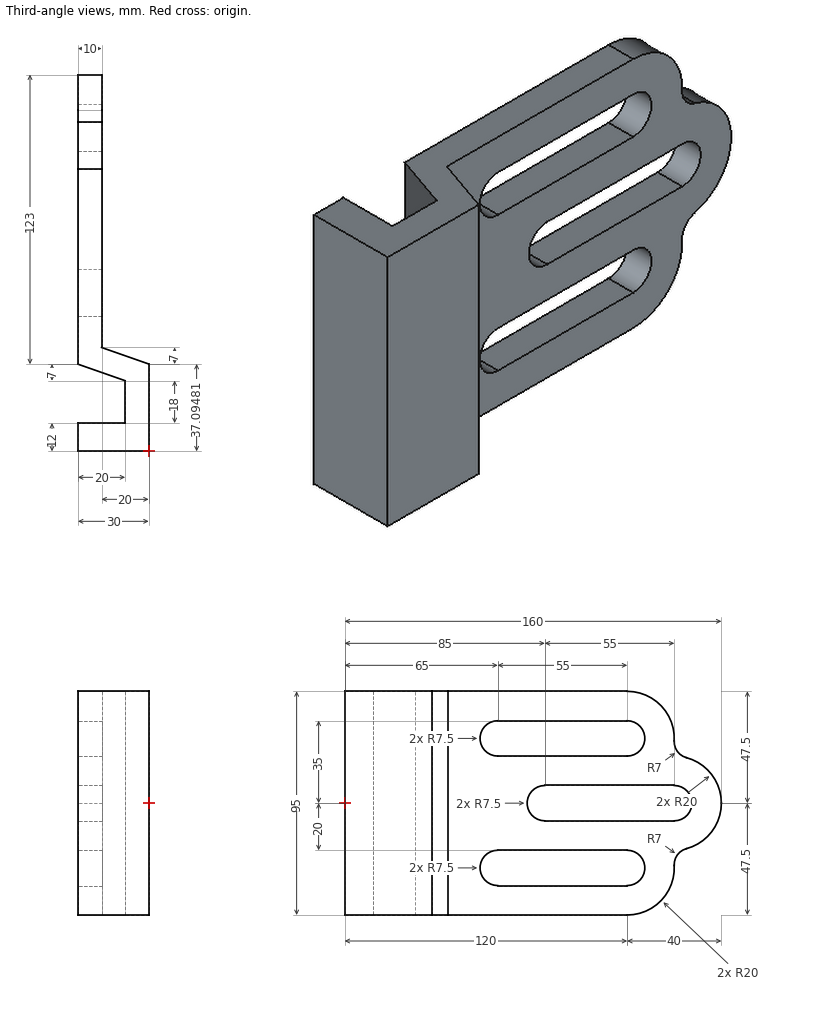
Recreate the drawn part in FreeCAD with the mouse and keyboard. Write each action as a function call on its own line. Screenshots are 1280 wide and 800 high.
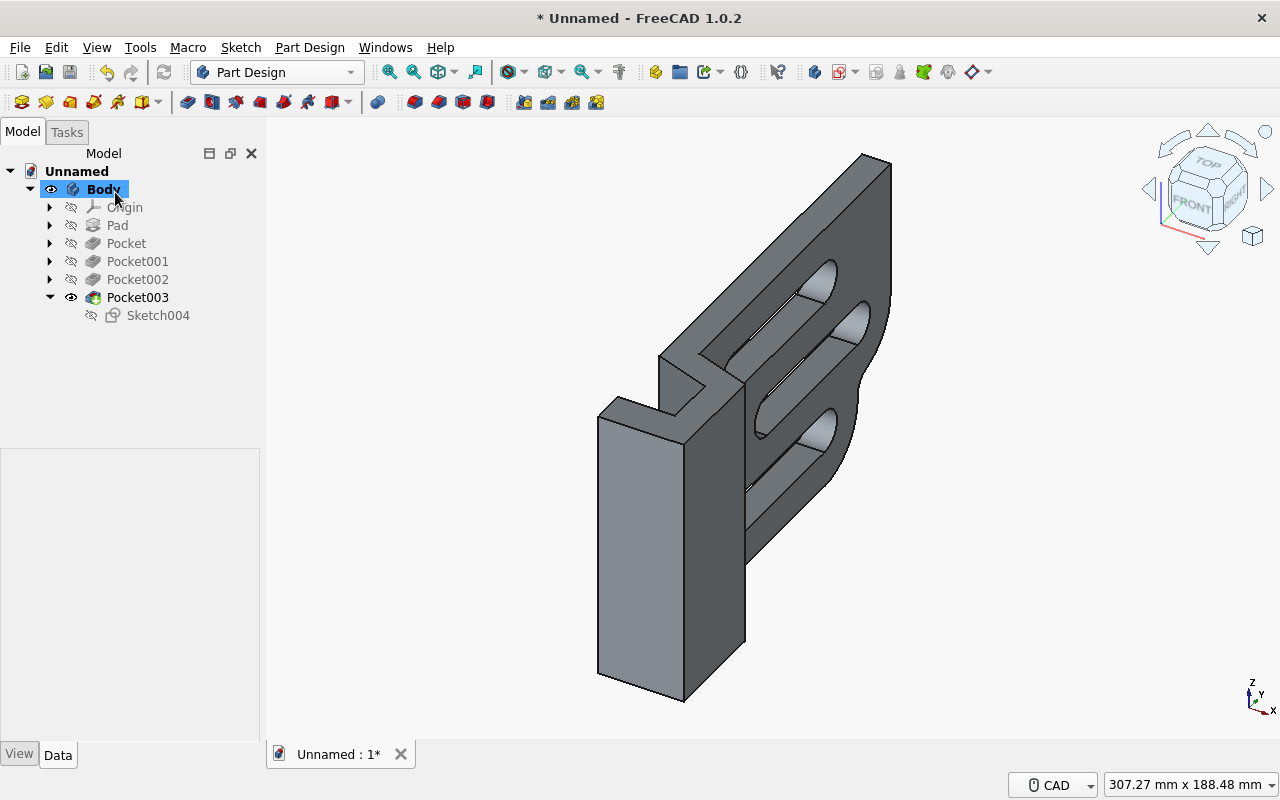
click(877, 231)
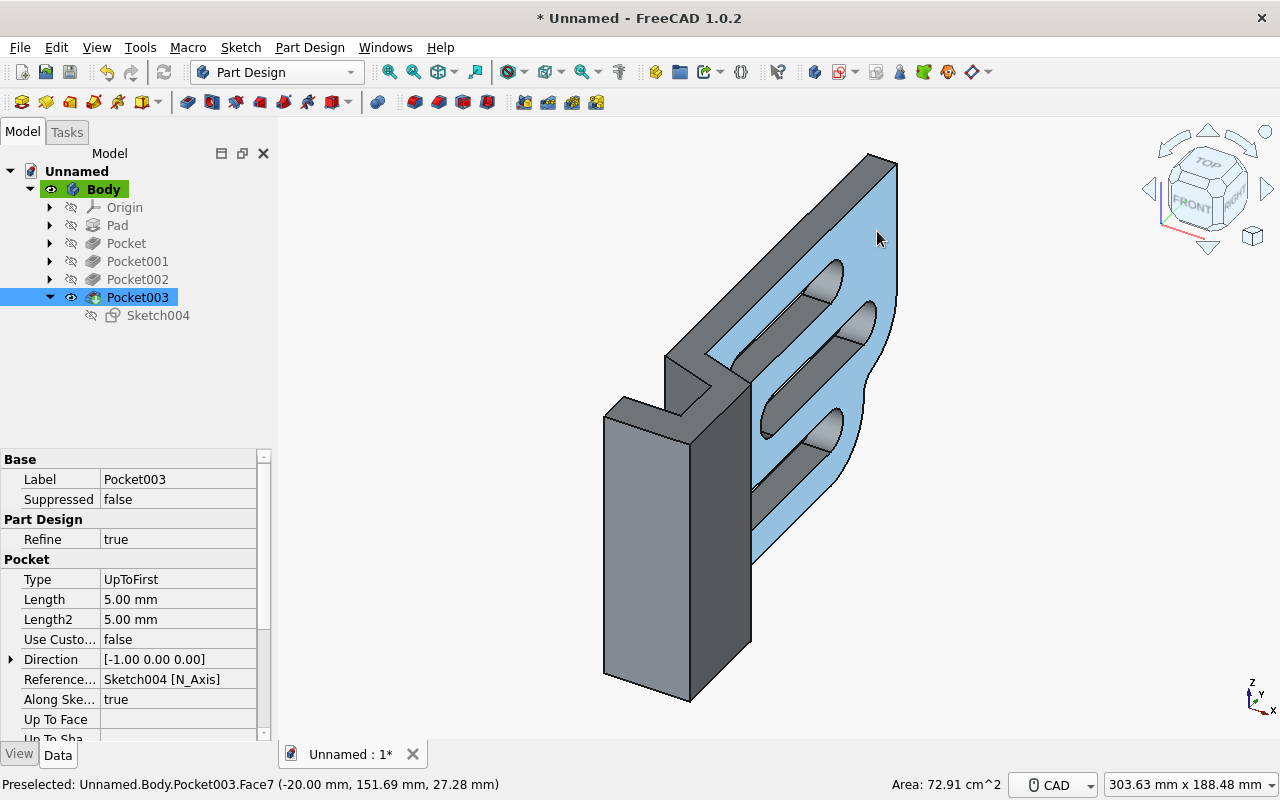
click(840, 72)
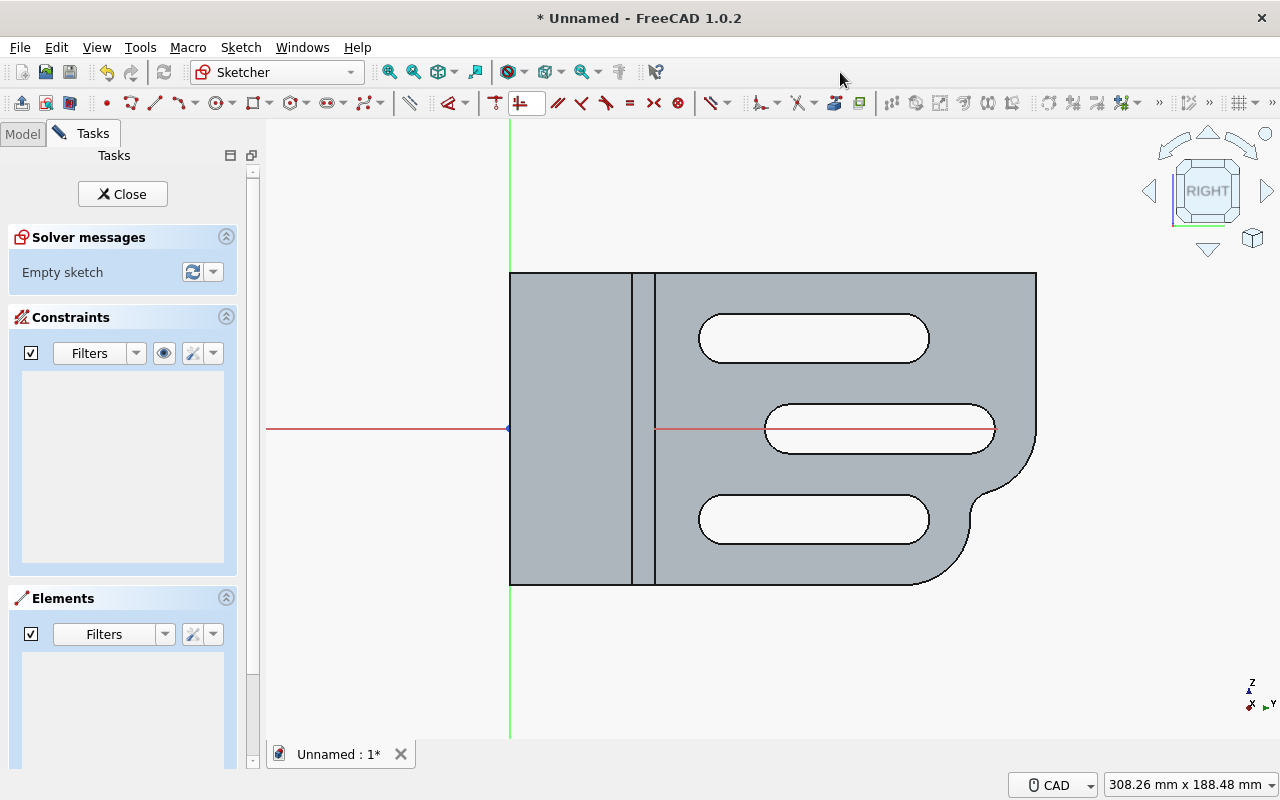
click(70, 104)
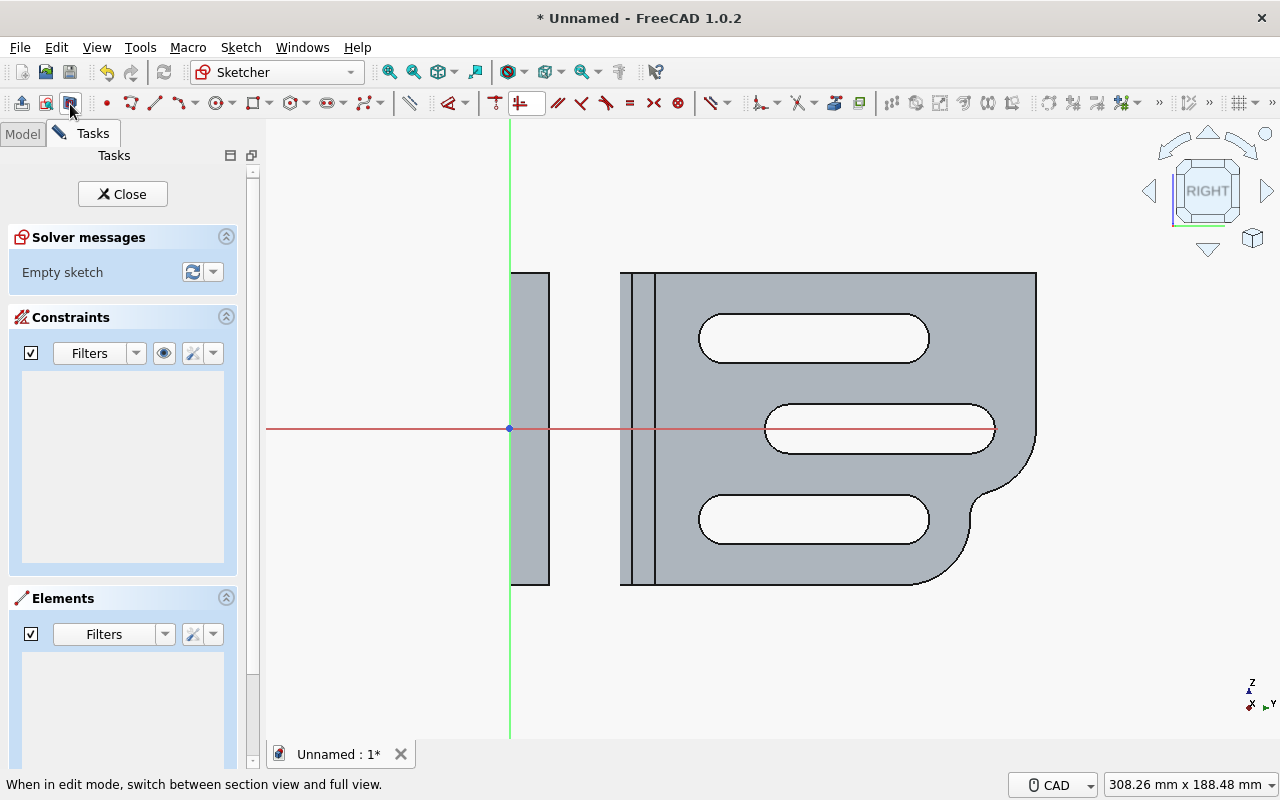
scroll(1115, 305, up, 5)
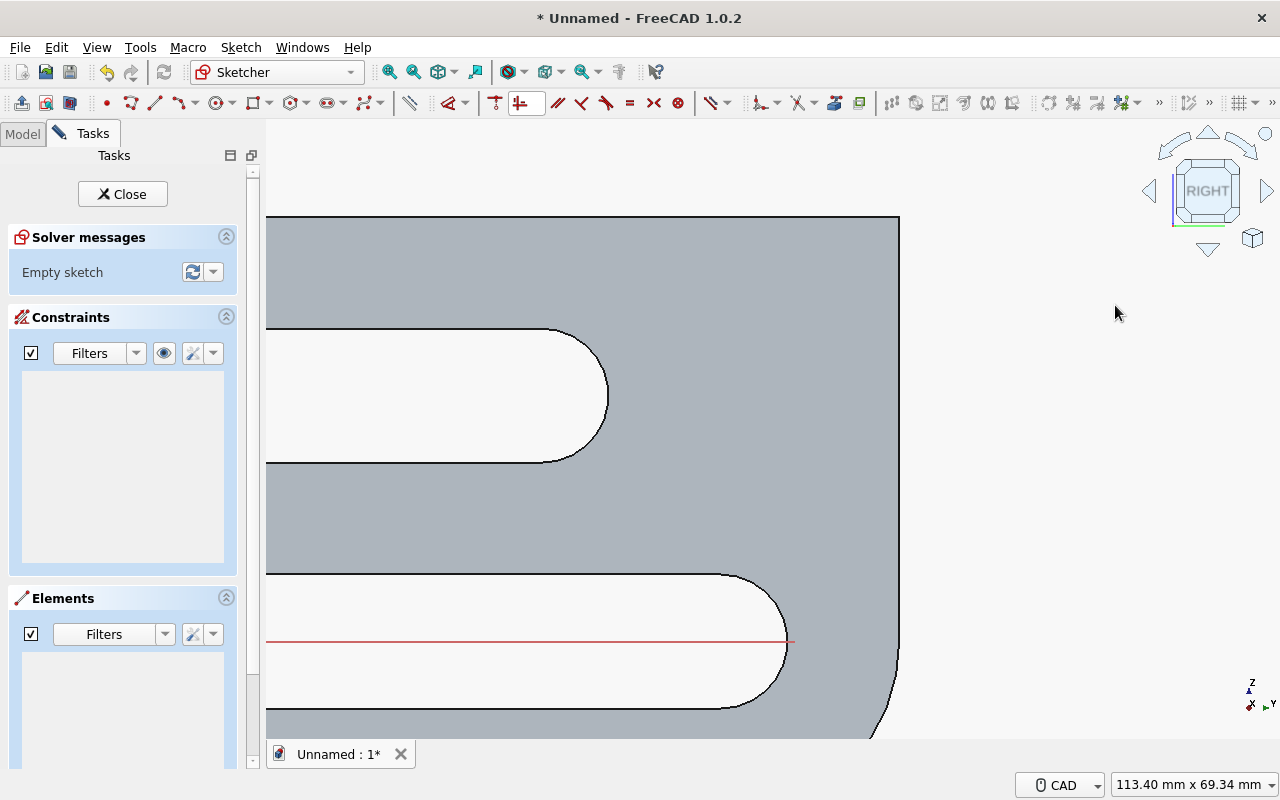
click(132, 104)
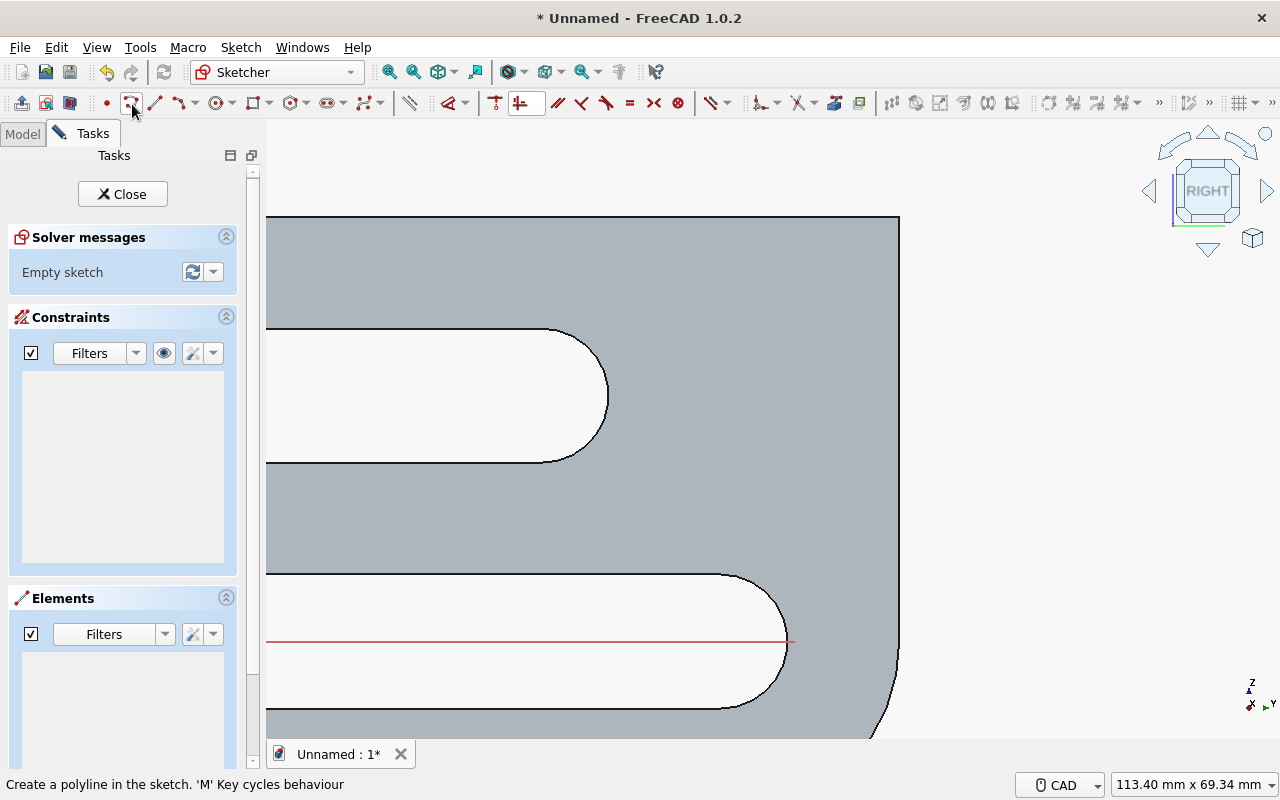
click(899, 642)
click(899, 217)
click(542, 217)
right_click(542, 217)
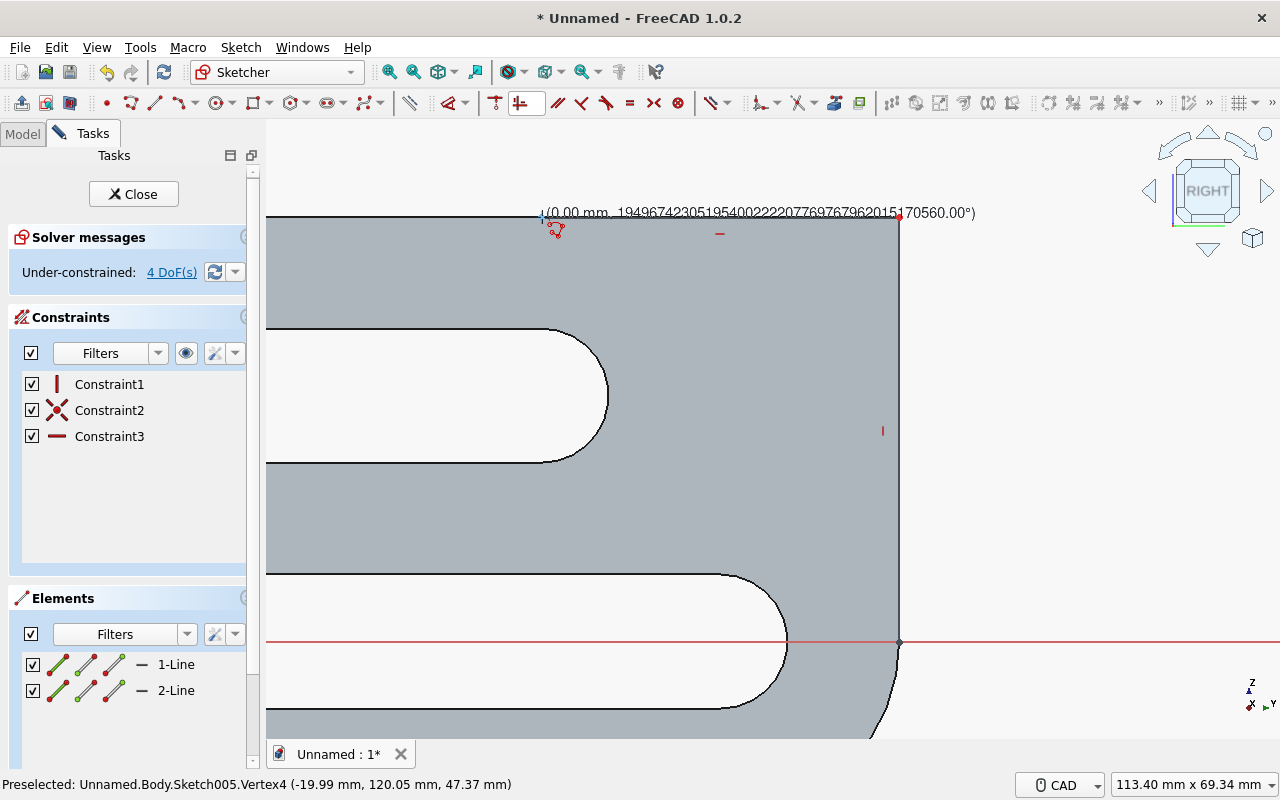
click(180, 104)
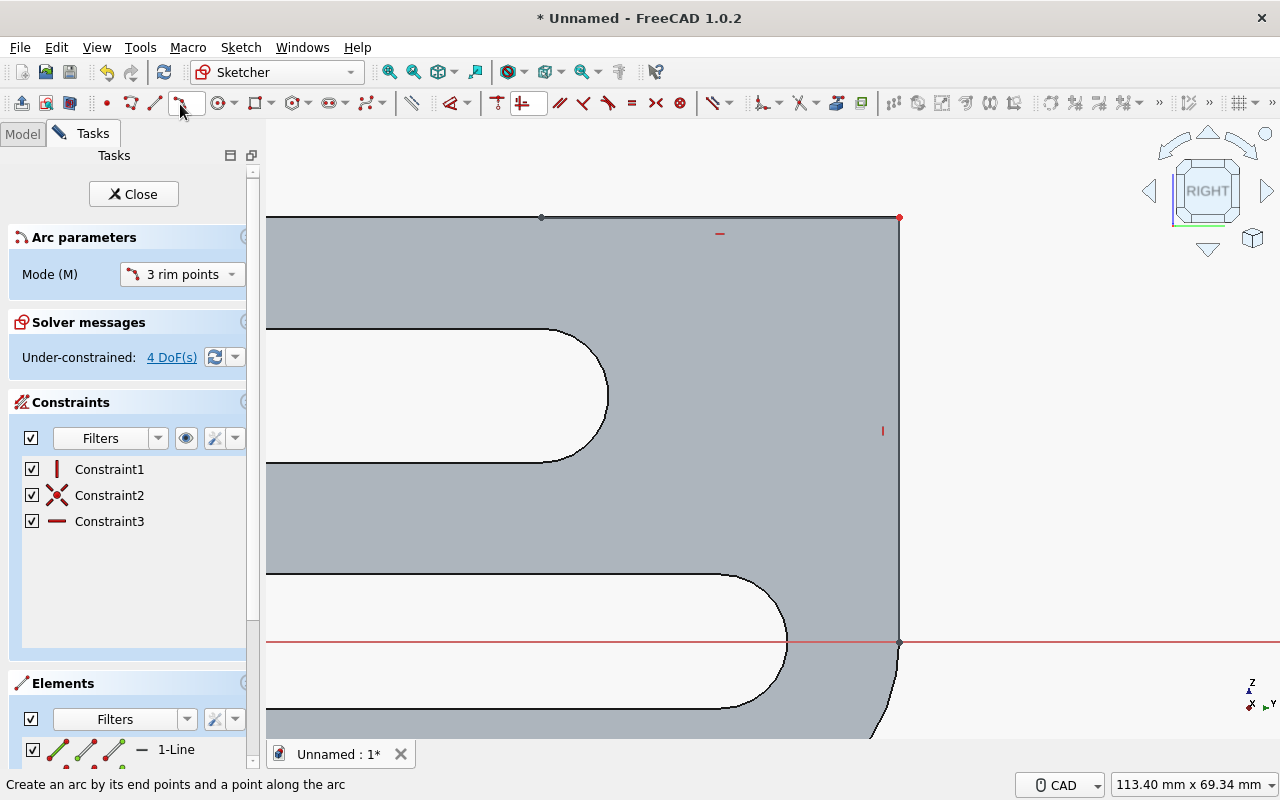
click(542, 218)
click(720, 405)
click(671, 273)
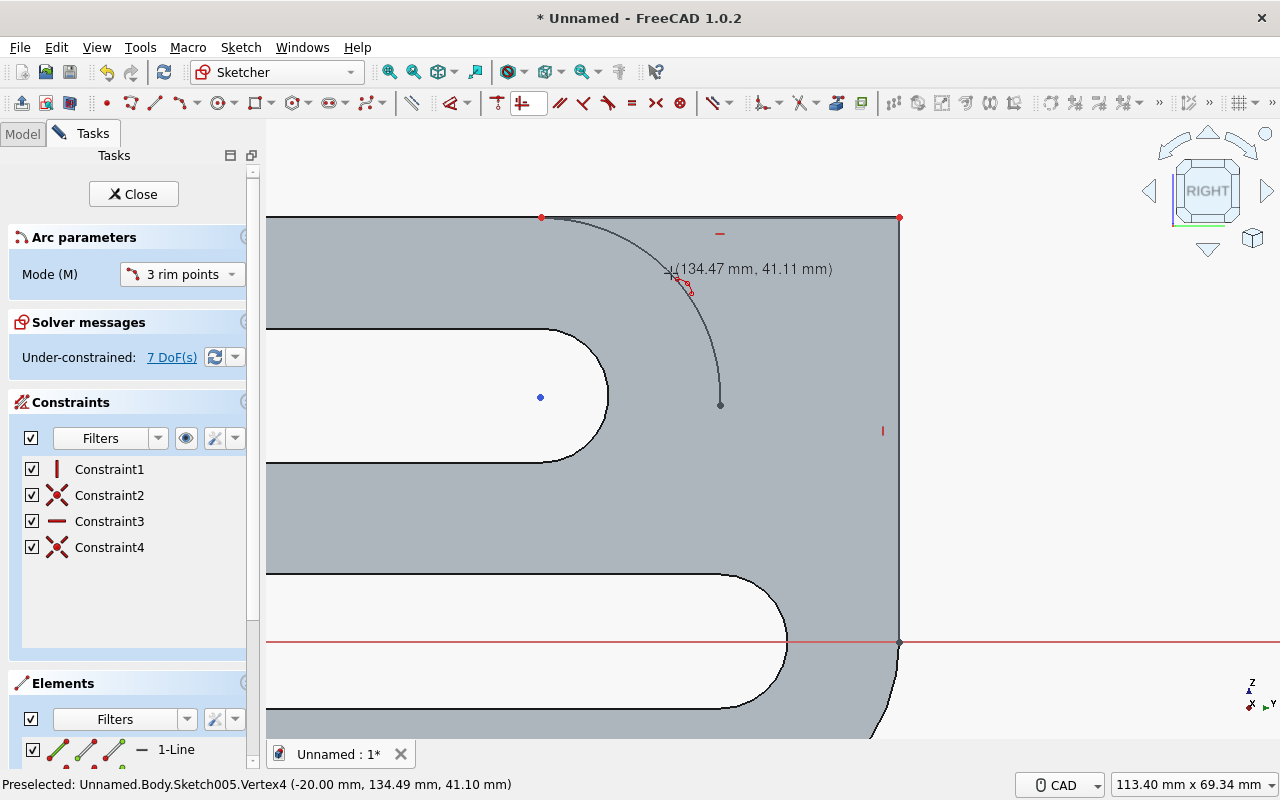
click(720, 406)
click(767, 469)
click(732, 445)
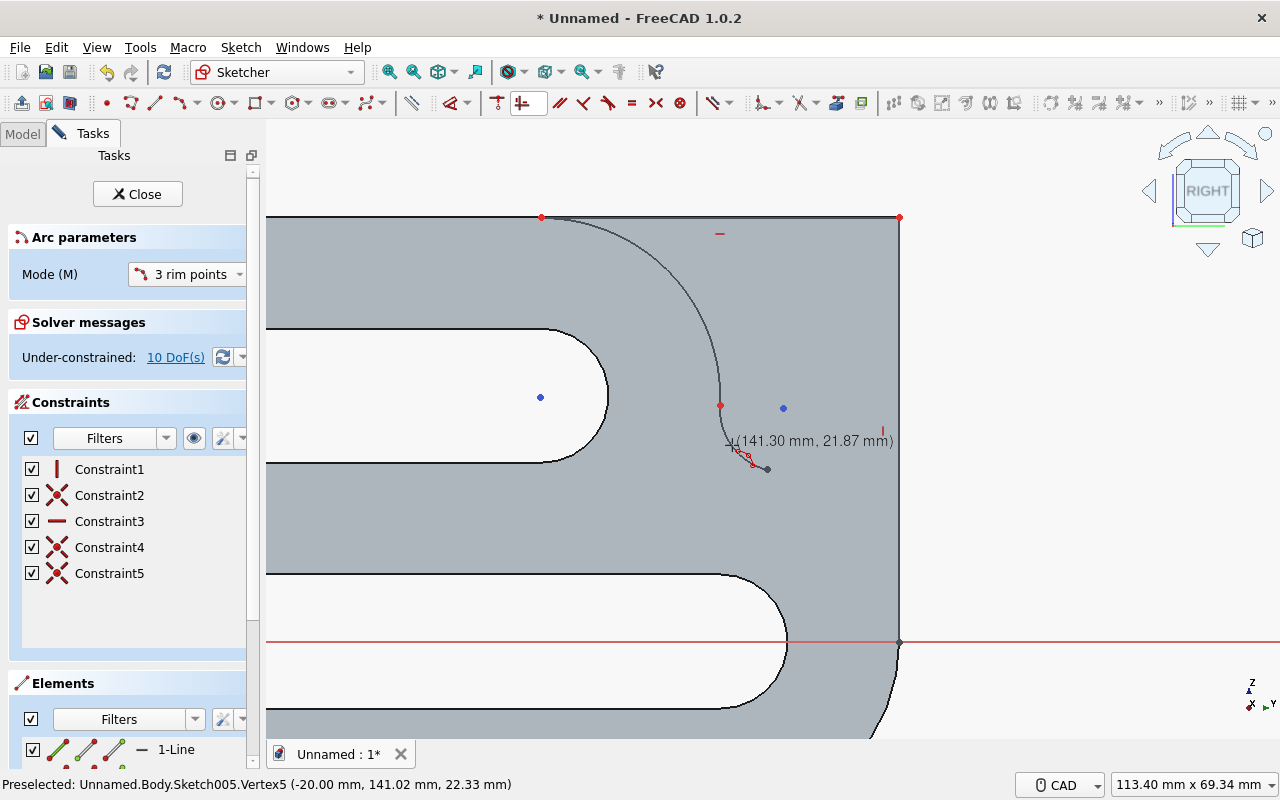
click(767, 470)
click(899, 643)
click(862, 533)
key(Escape)